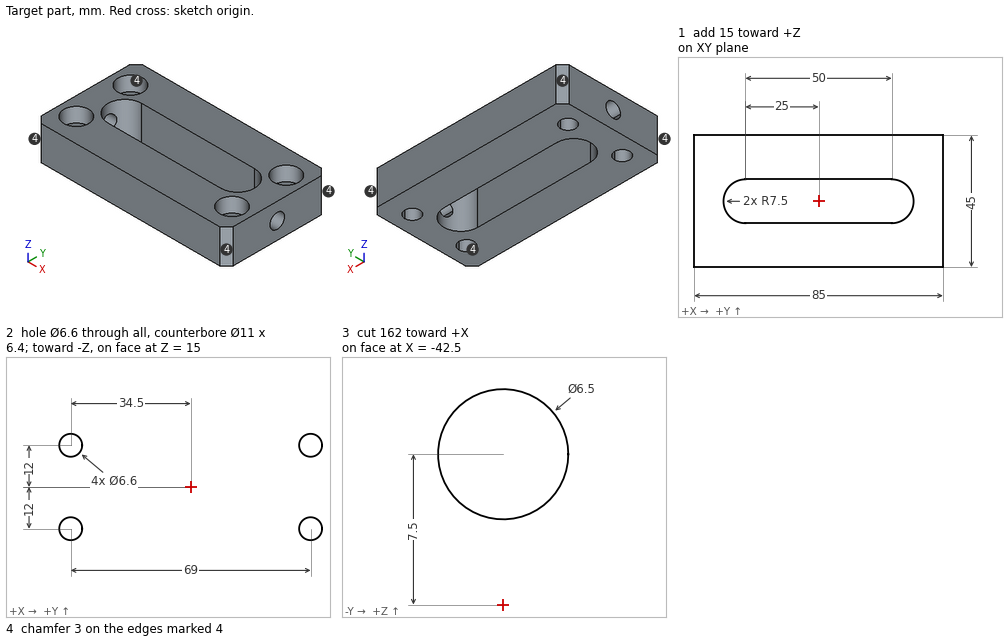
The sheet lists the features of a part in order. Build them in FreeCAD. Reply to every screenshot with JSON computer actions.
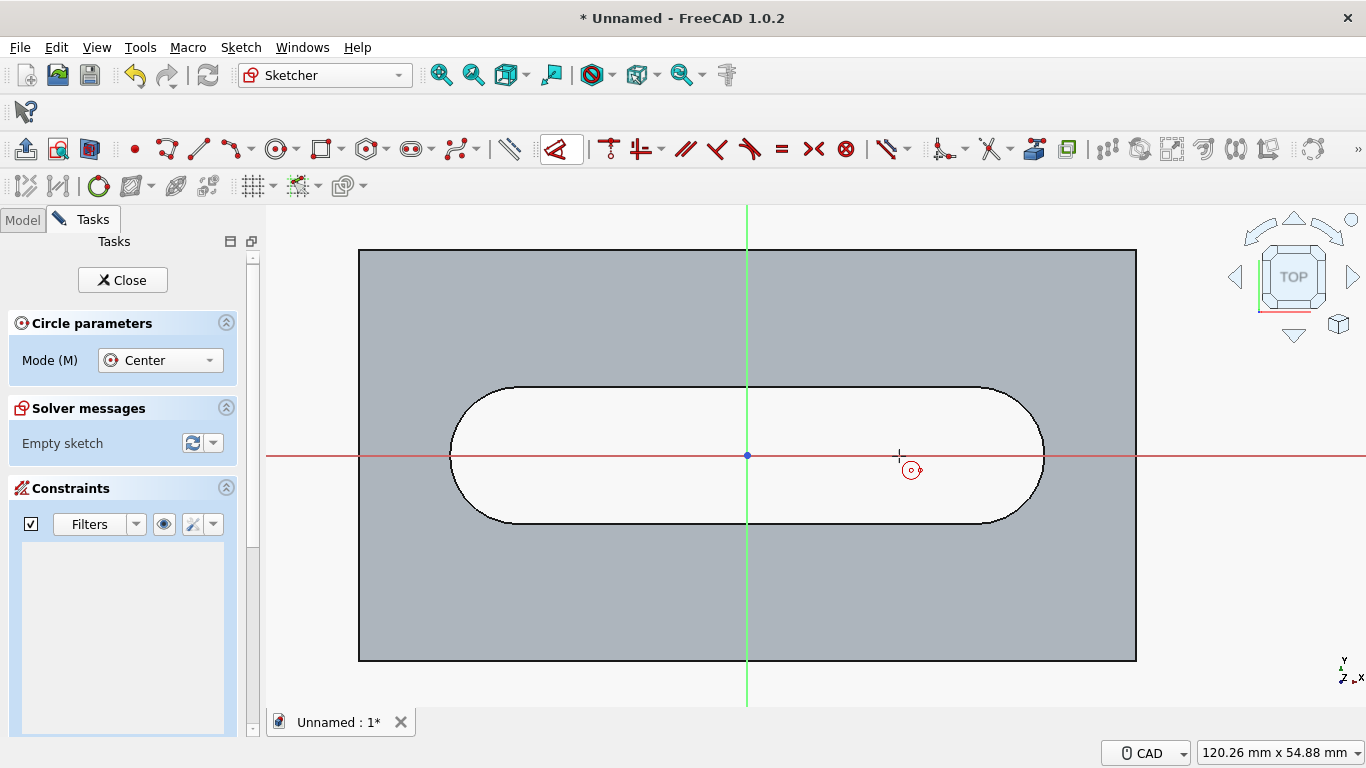
{"action": "left_click", "coordinate": [432, 346]}
{"action": "left_click", "coordinate": [453, 324]}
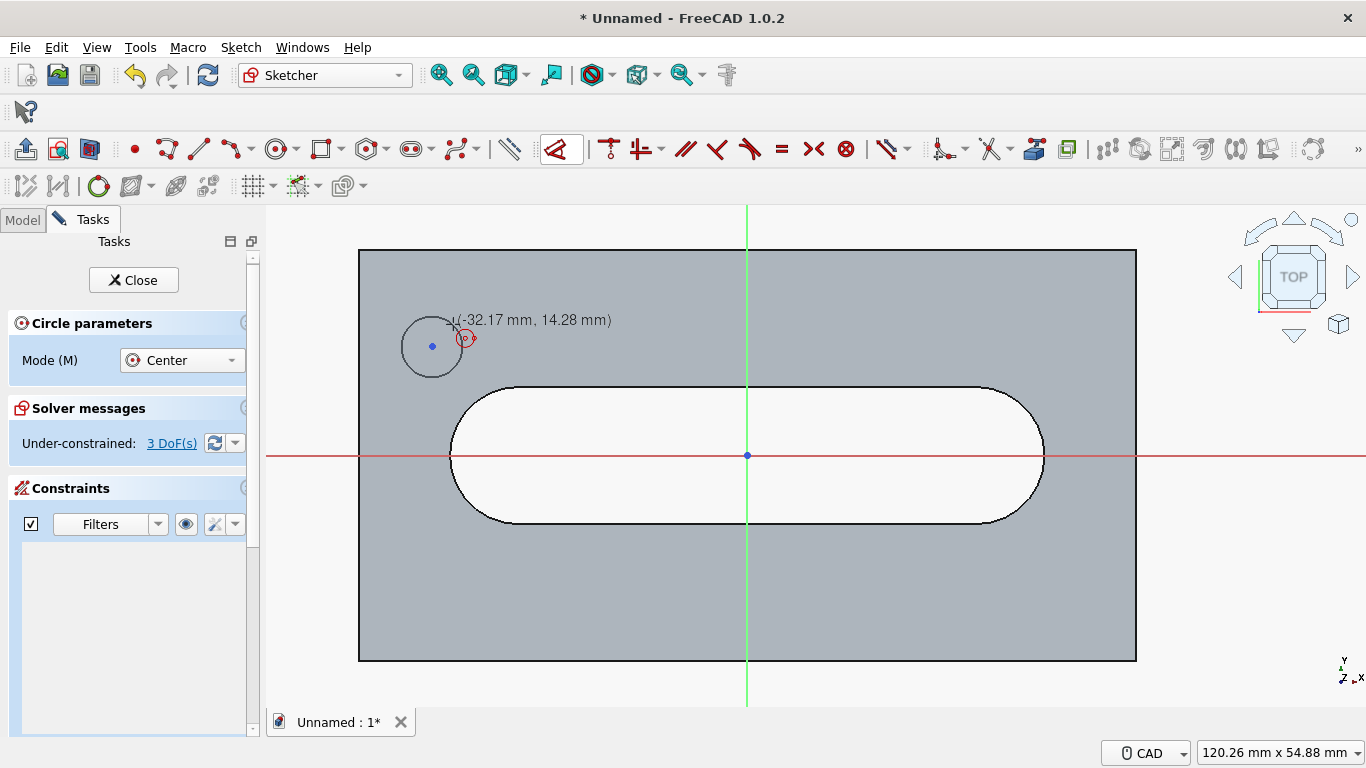
{"action": "left_click", "coordinate": [432, 565]}
{"action": "left_click", "coordinate": [453, 544]}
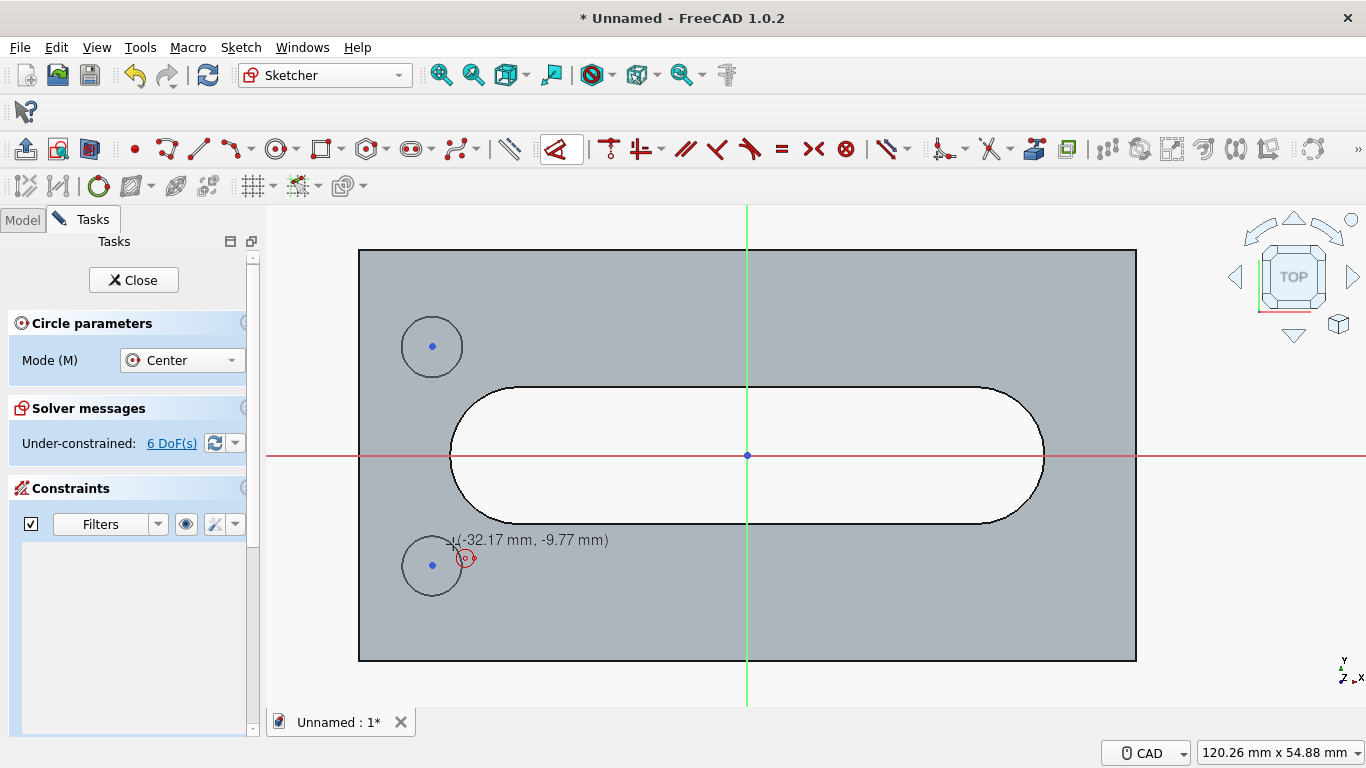
{"action": "left_click", "coordinate": [1063, 565]}
{"action": "left_click", "coordinate": [1084, 544]}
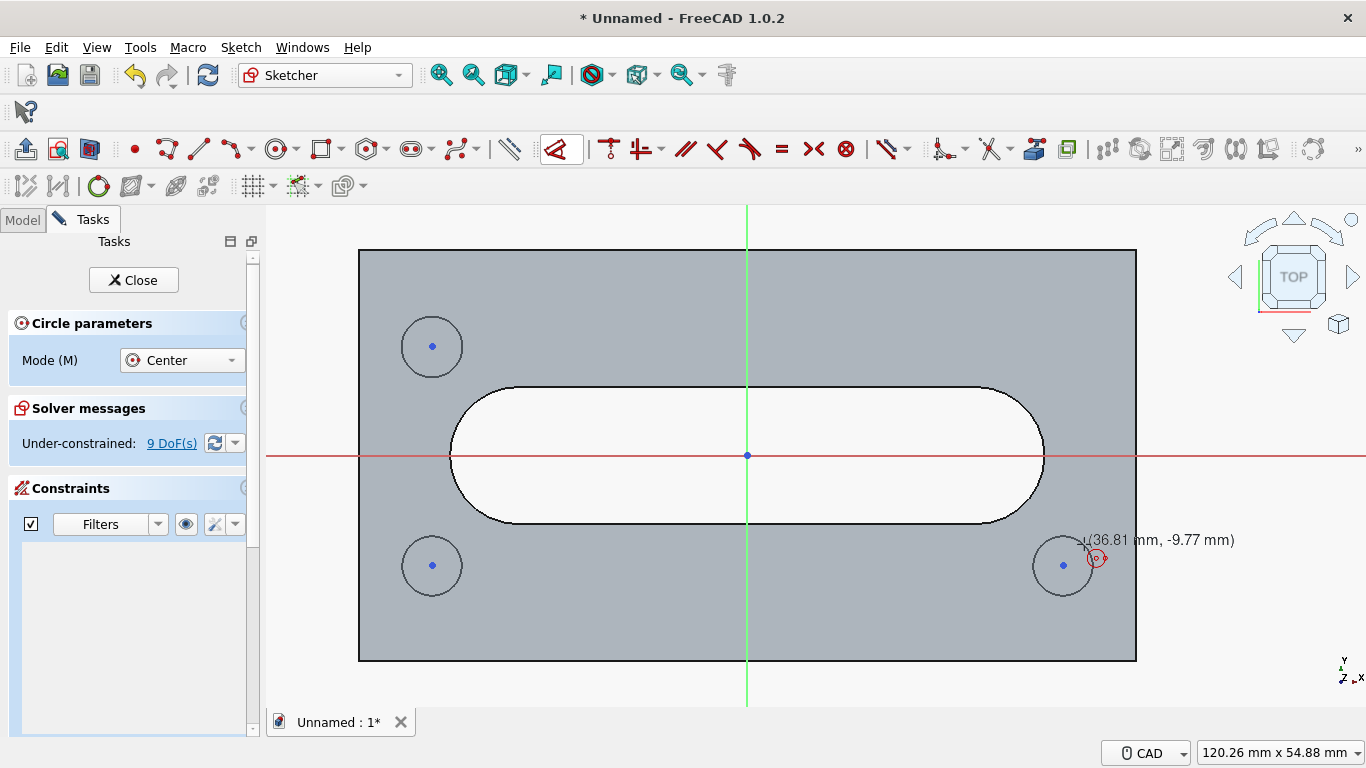
{"action": "left_click", "coordinate": [1063, 346]}
{"action": "left_click", "coordinate": [1084, 324]}
{"action": "key", "text": "Escape"}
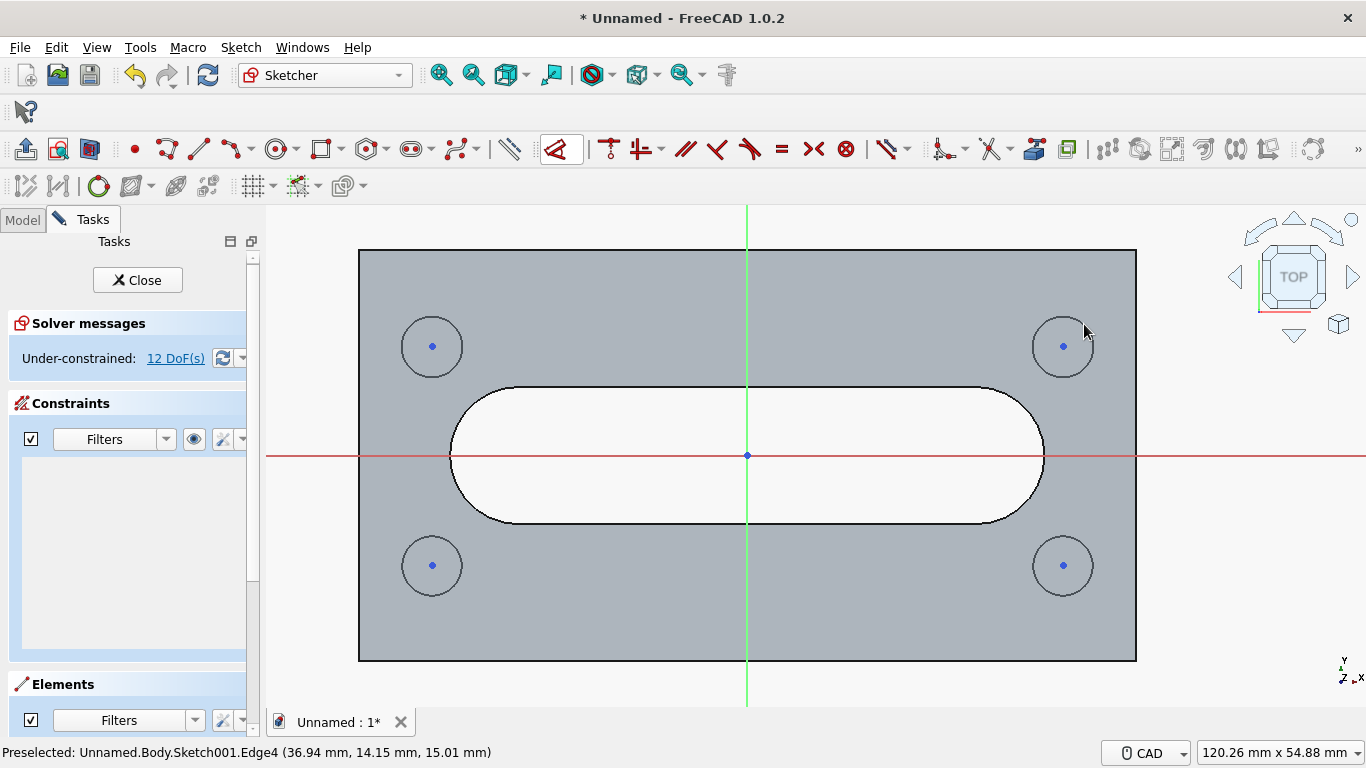
{"action": "left_click", "coordinate": [453, 325]}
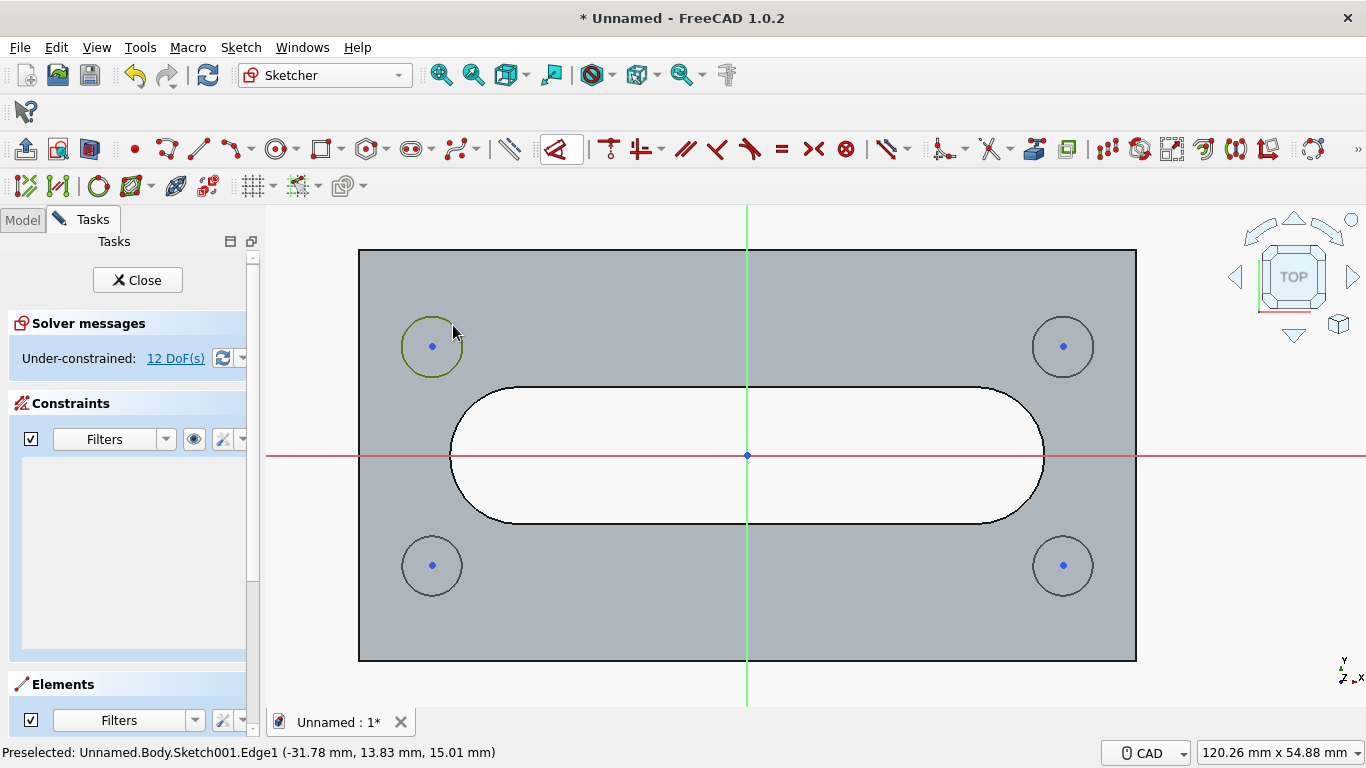
{"action": "left_click", "coordinate": [453, 545]}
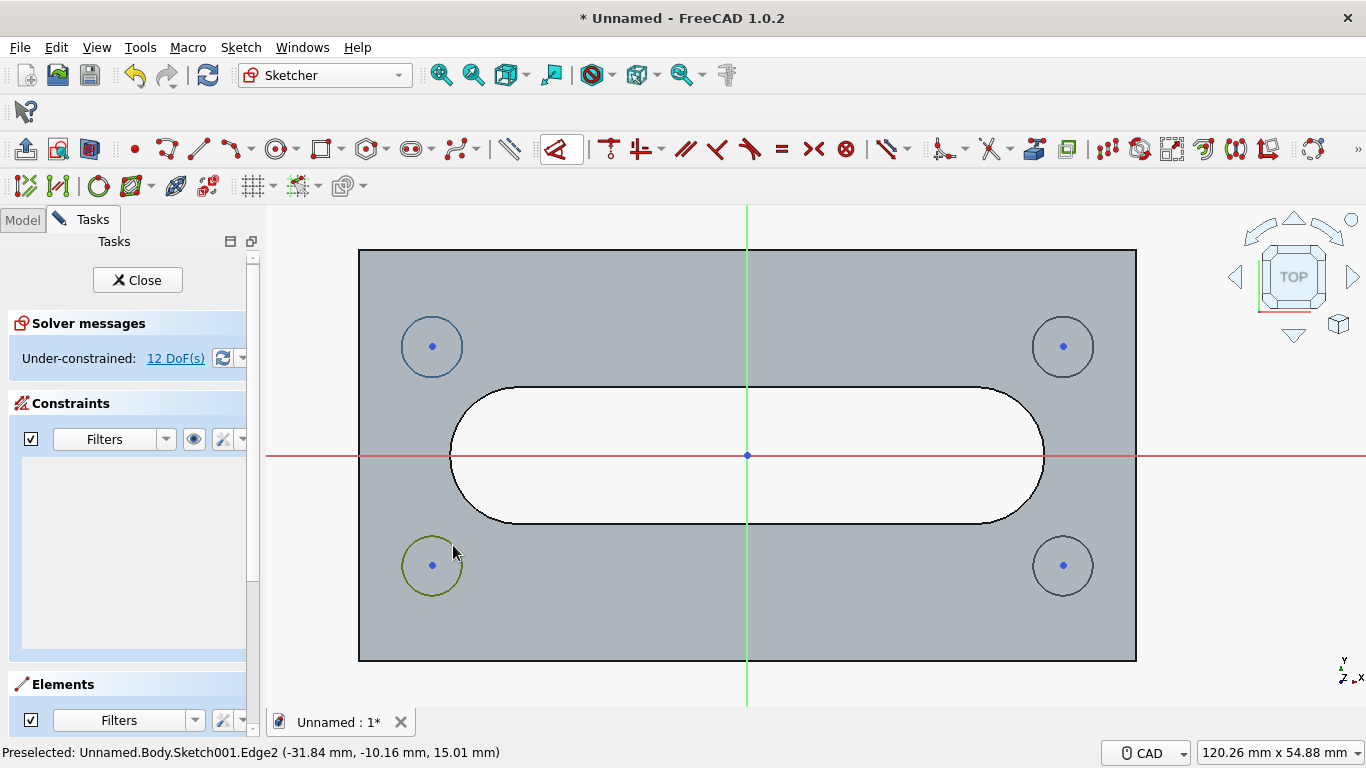
{"action": "left_click", "coordinate": [1084, 545]}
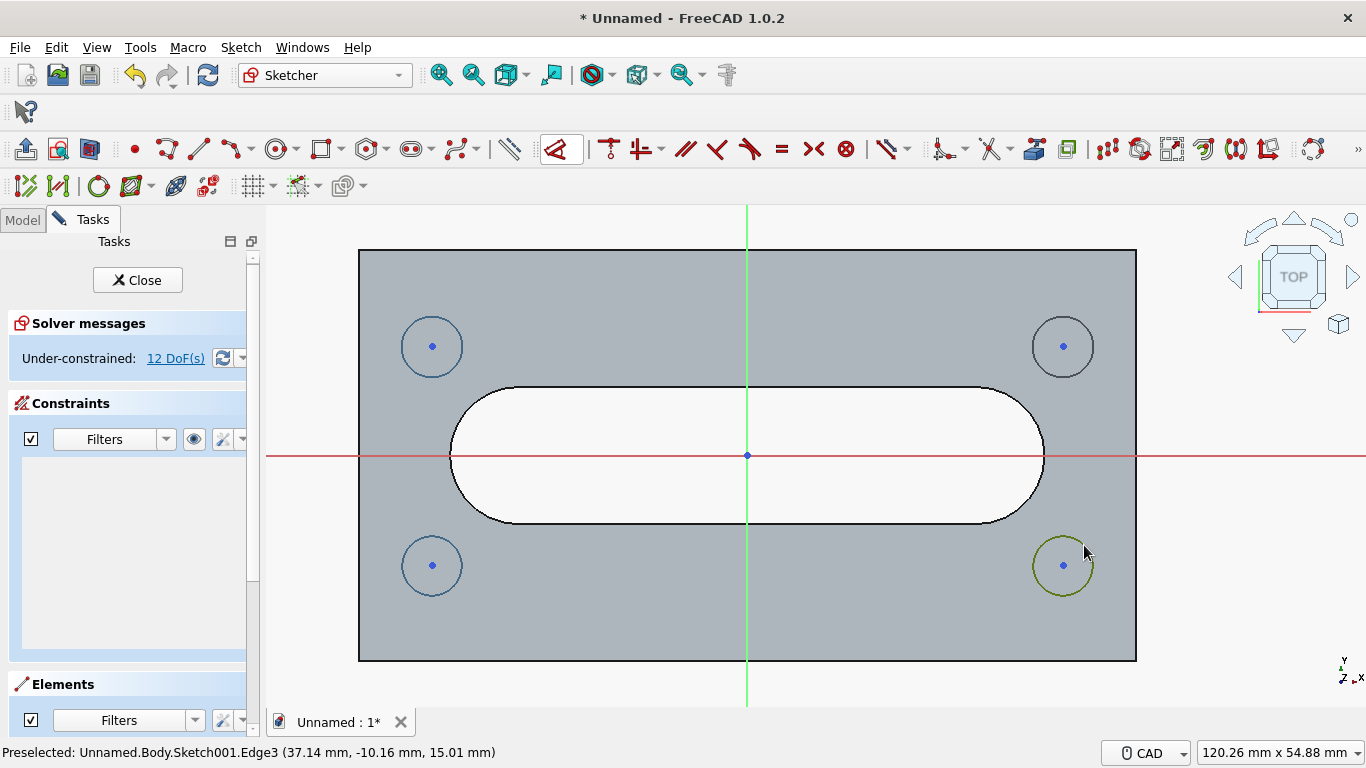
{"action": "left_click", "coordinate": [1084, 325]}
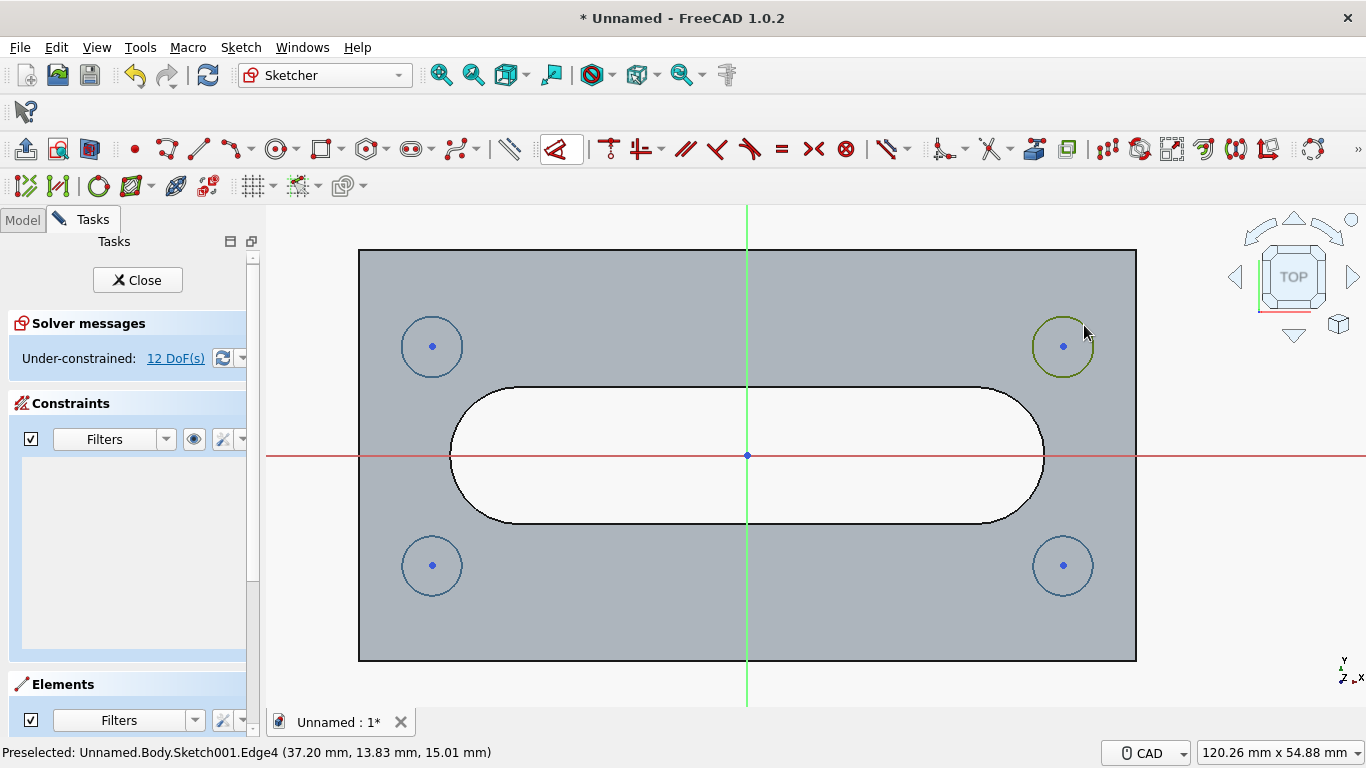
{"action": "left_click", "coordinate": [782, 150]}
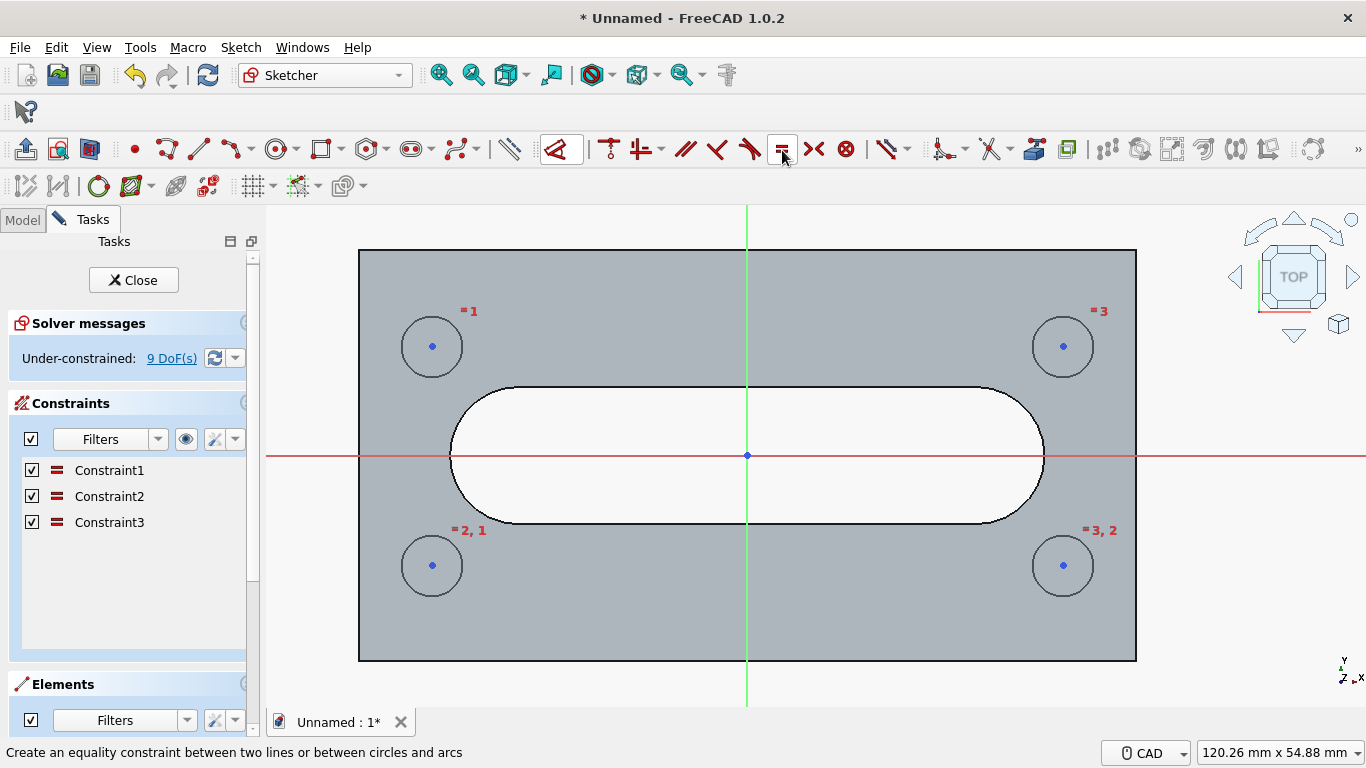
{"action": "left_click", "coordinate": [432, 347]}